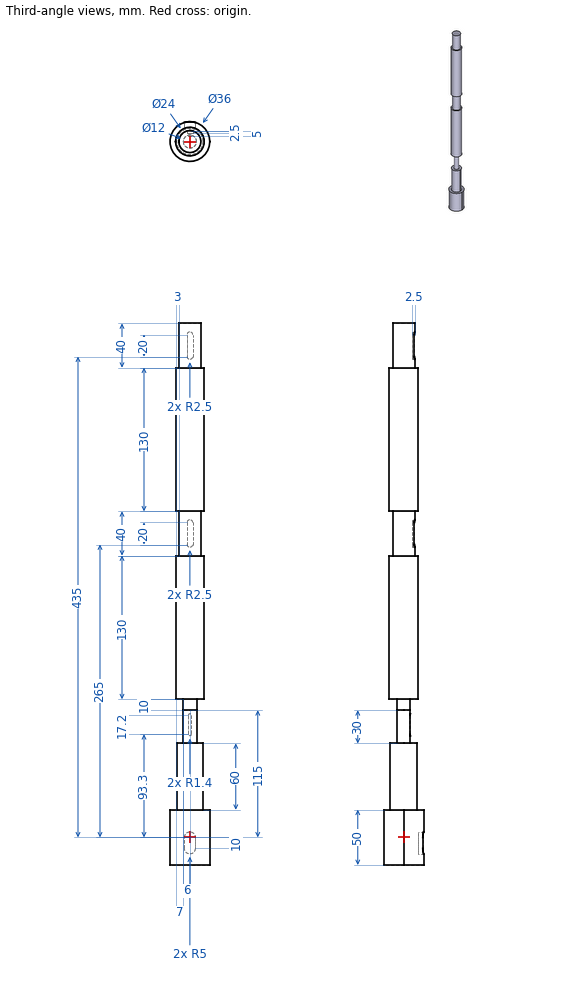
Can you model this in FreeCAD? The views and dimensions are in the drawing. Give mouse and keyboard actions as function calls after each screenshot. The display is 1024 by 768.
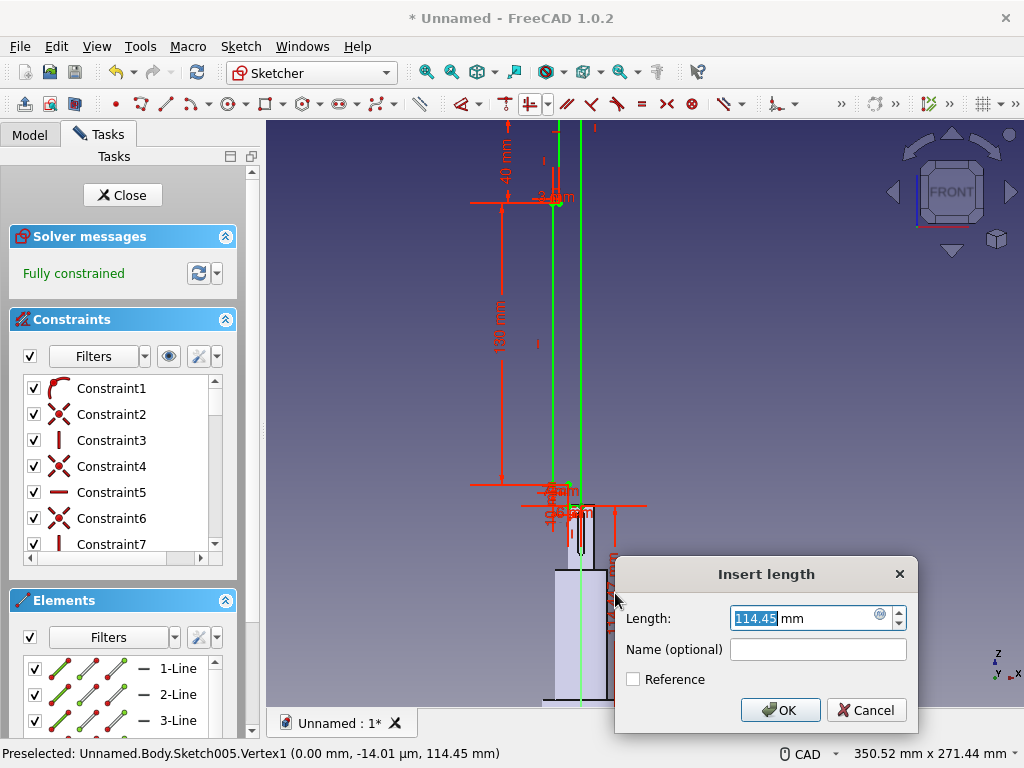
text(115)
key(Return)
key(Escape)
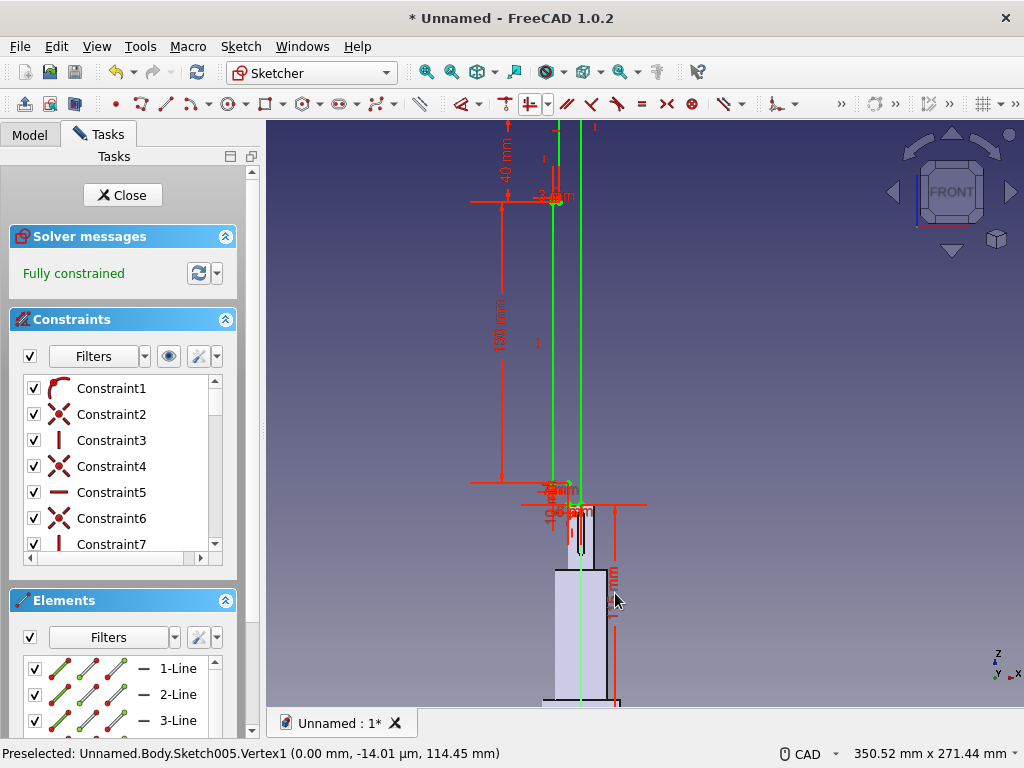
click(123, 195)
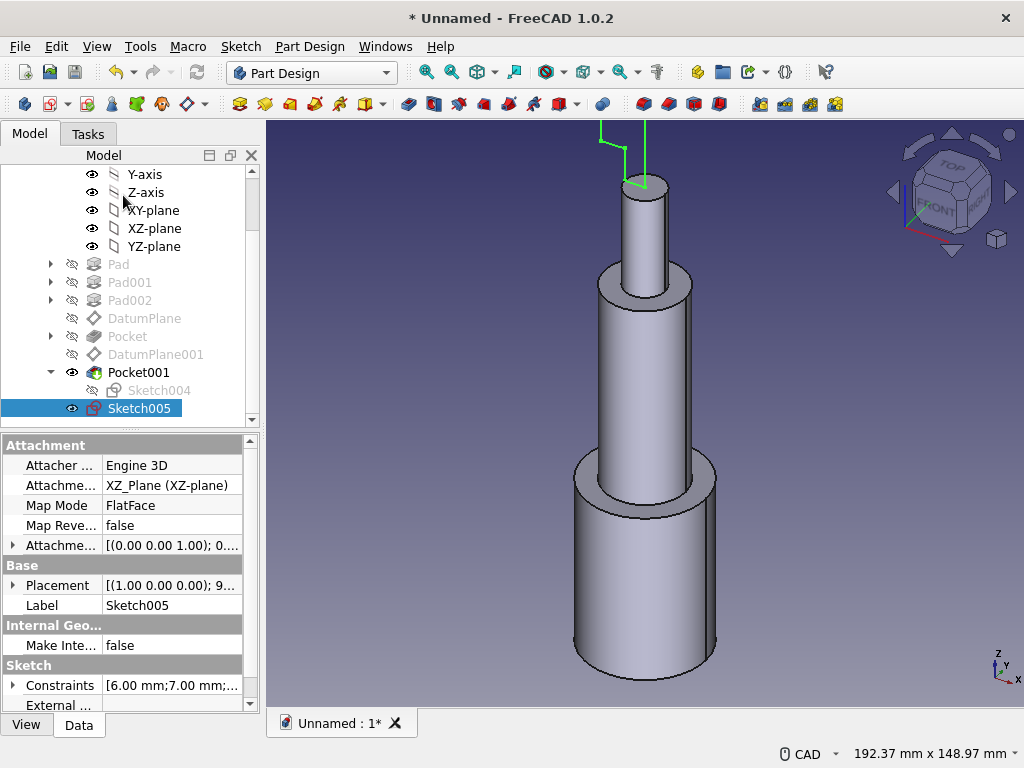
click(265, 104)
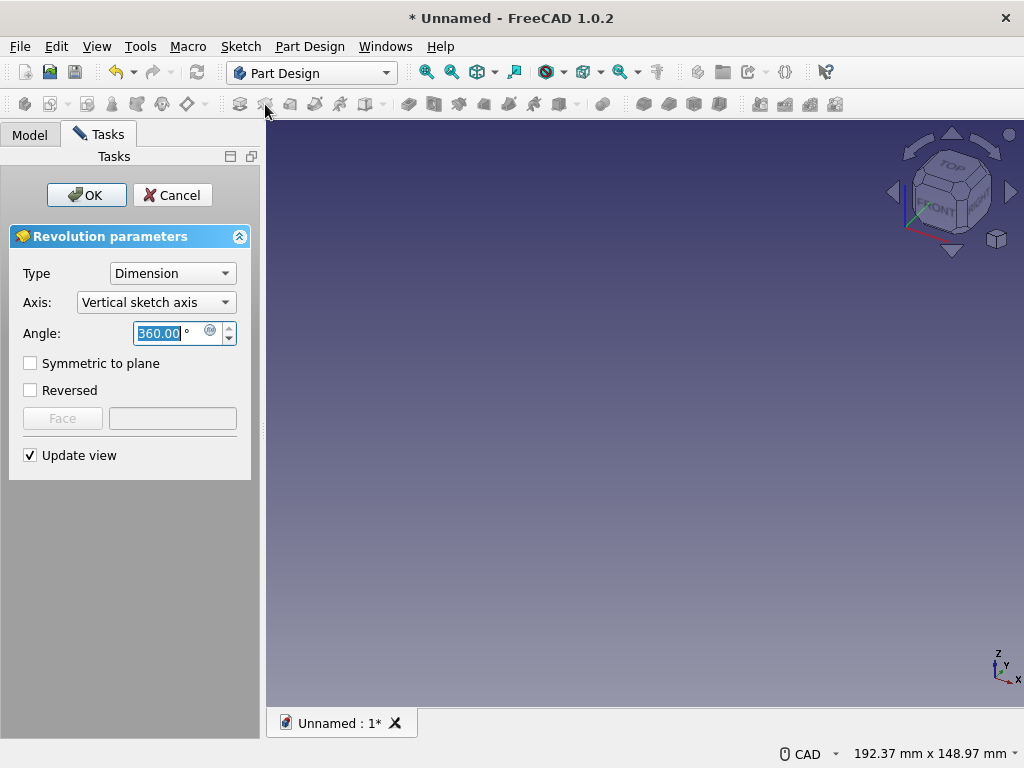
click(87, 195)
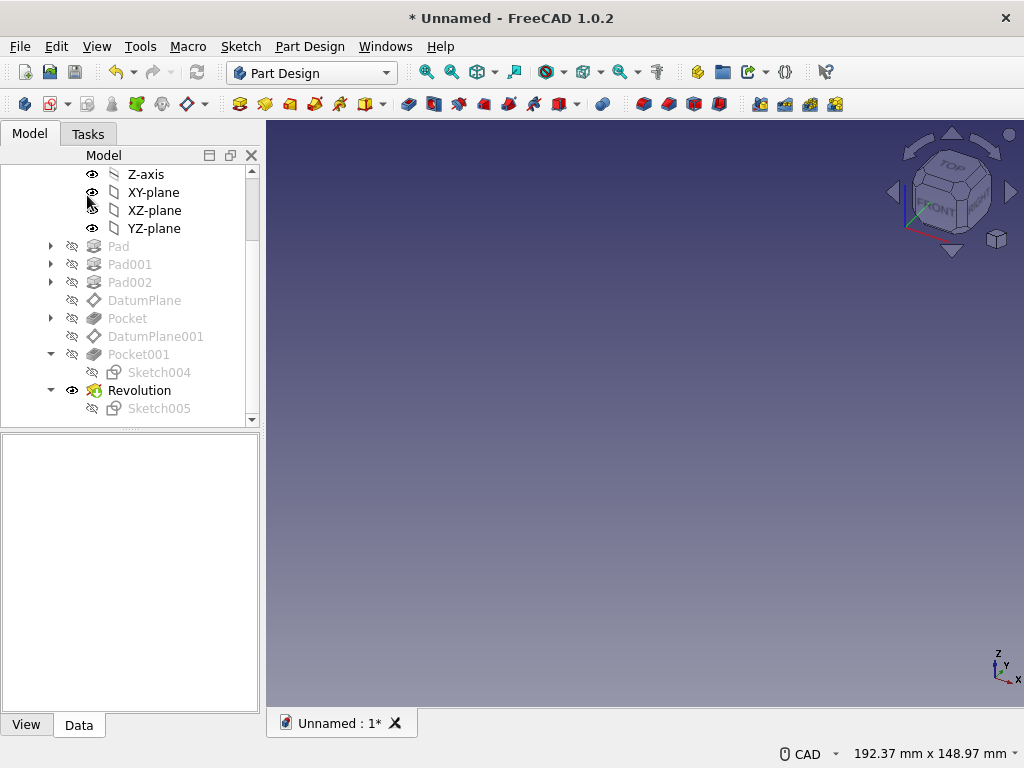
click(427, 72)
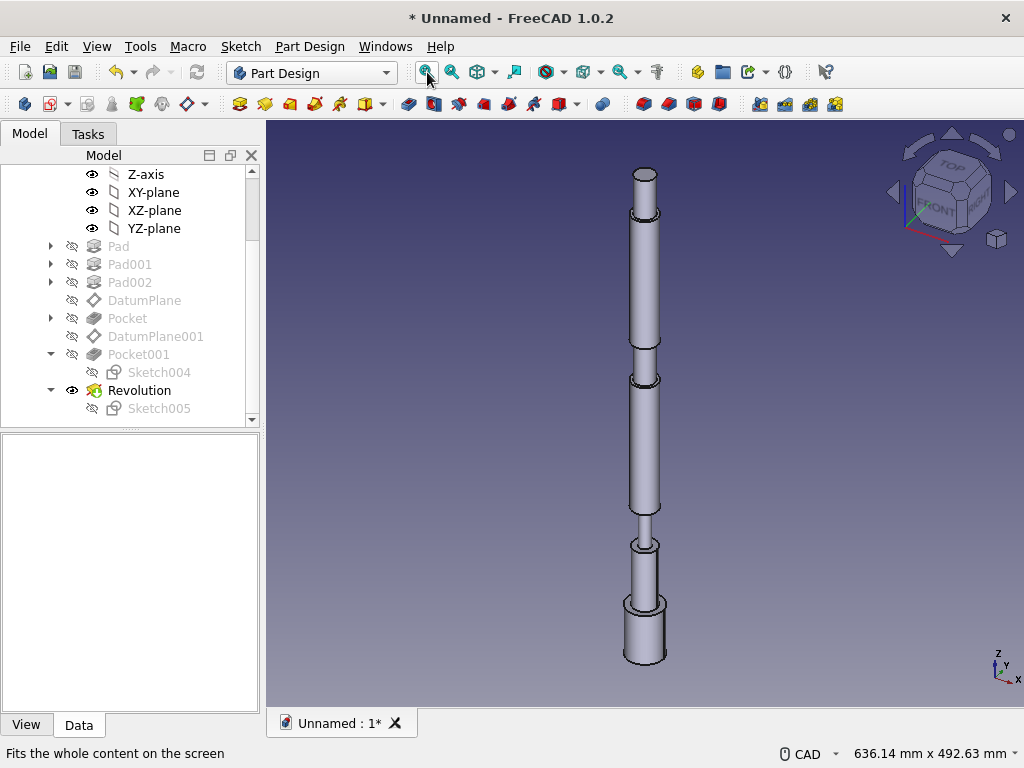
scroll(161, 296, down, 3)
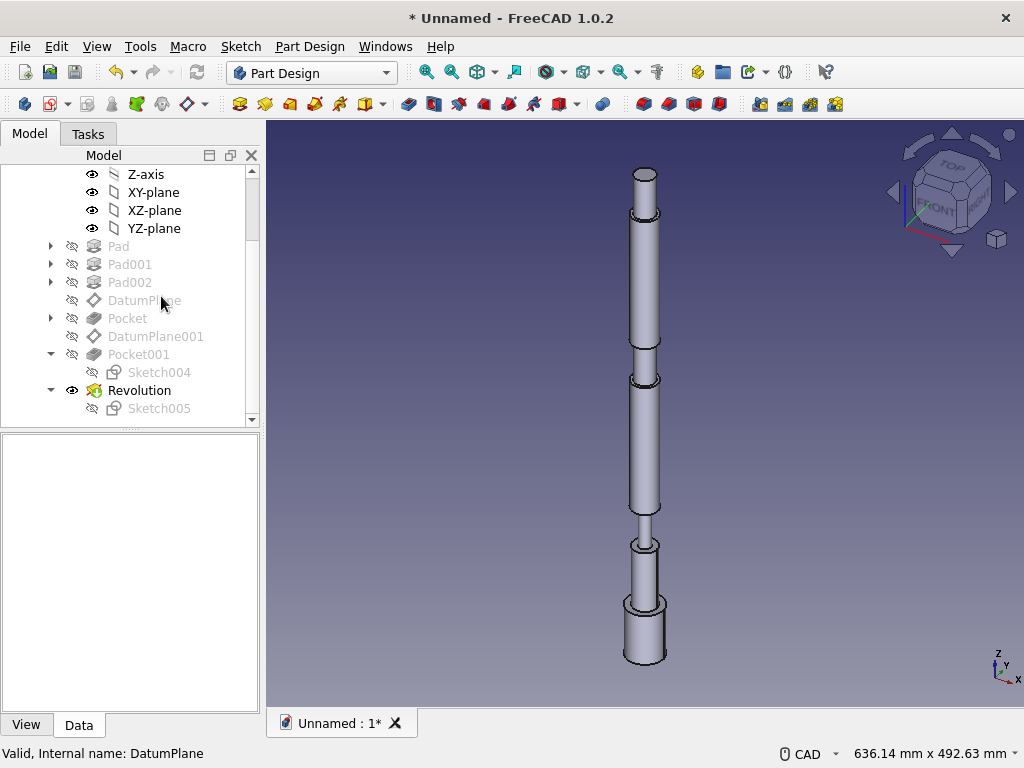
scroll(161, 296, up, 15)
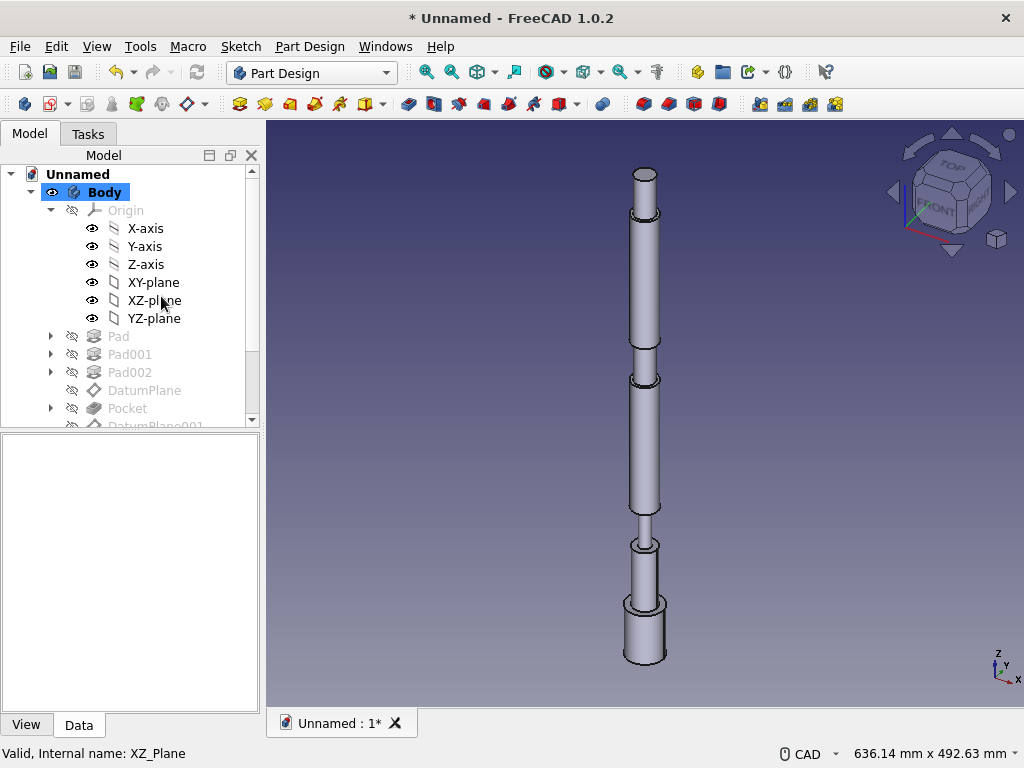
click(137, 300)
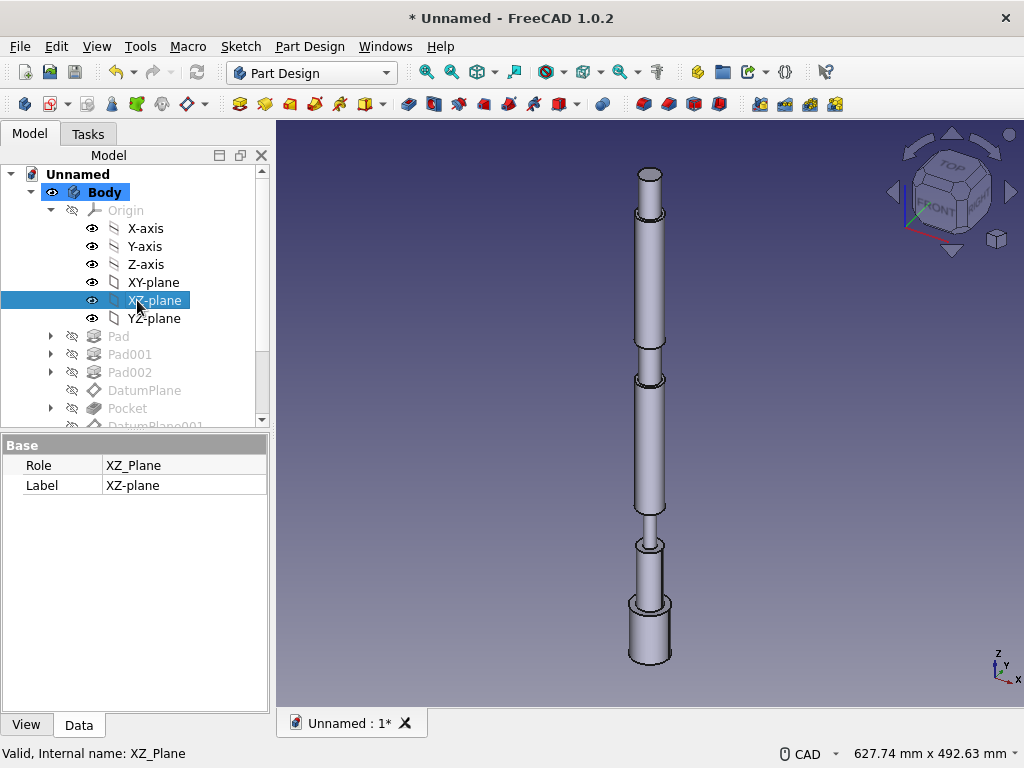
click(186, 104)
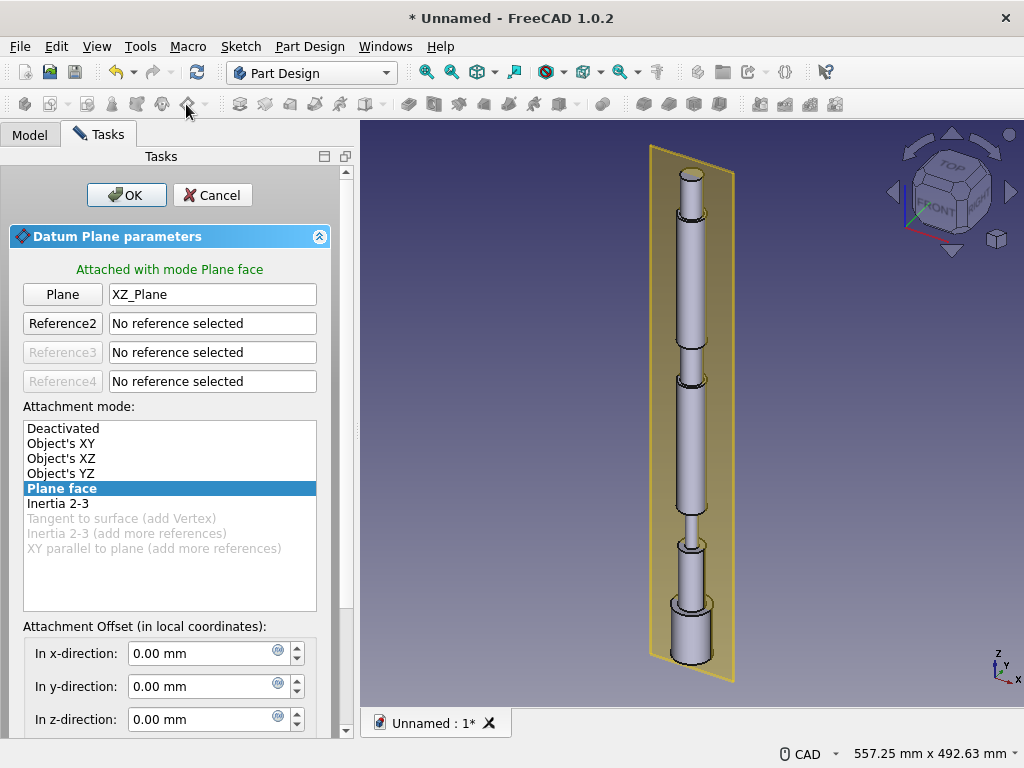
triple_click(210, 720)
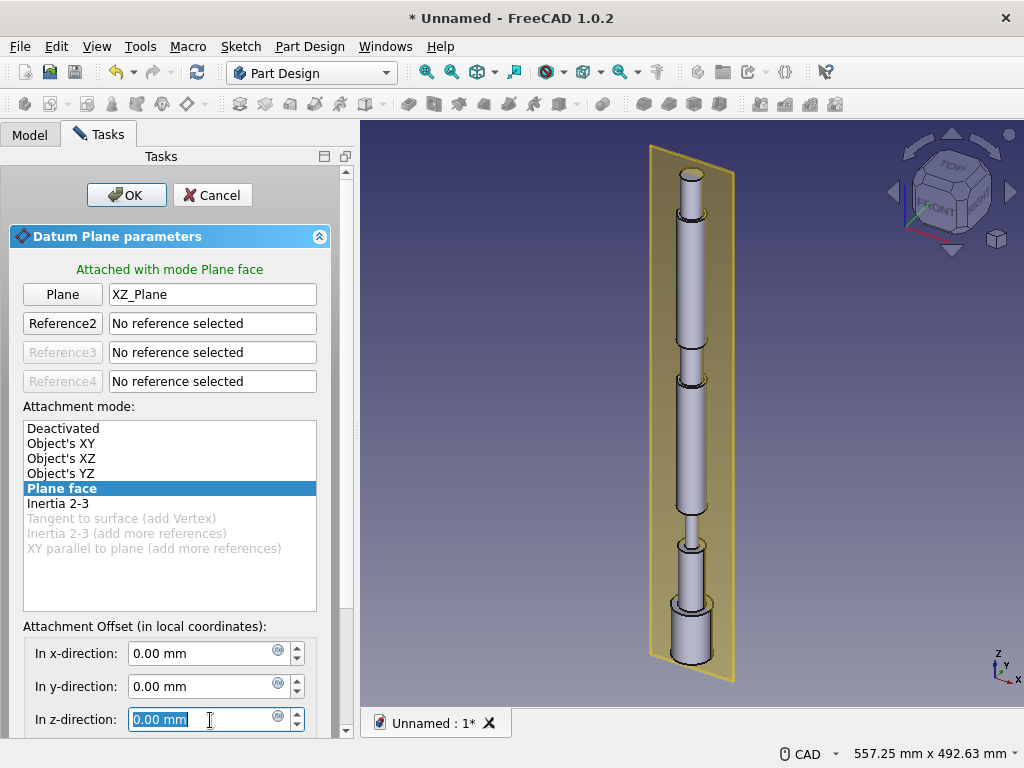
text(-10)
key(Tab)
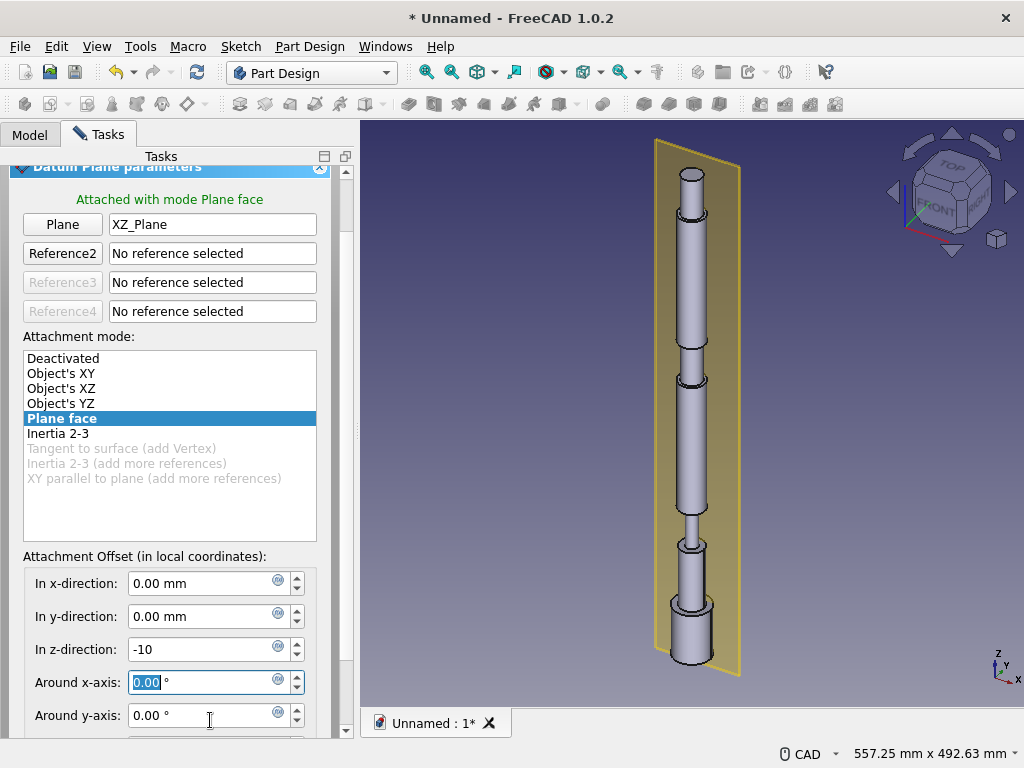
scroll(346, 452, up, 2)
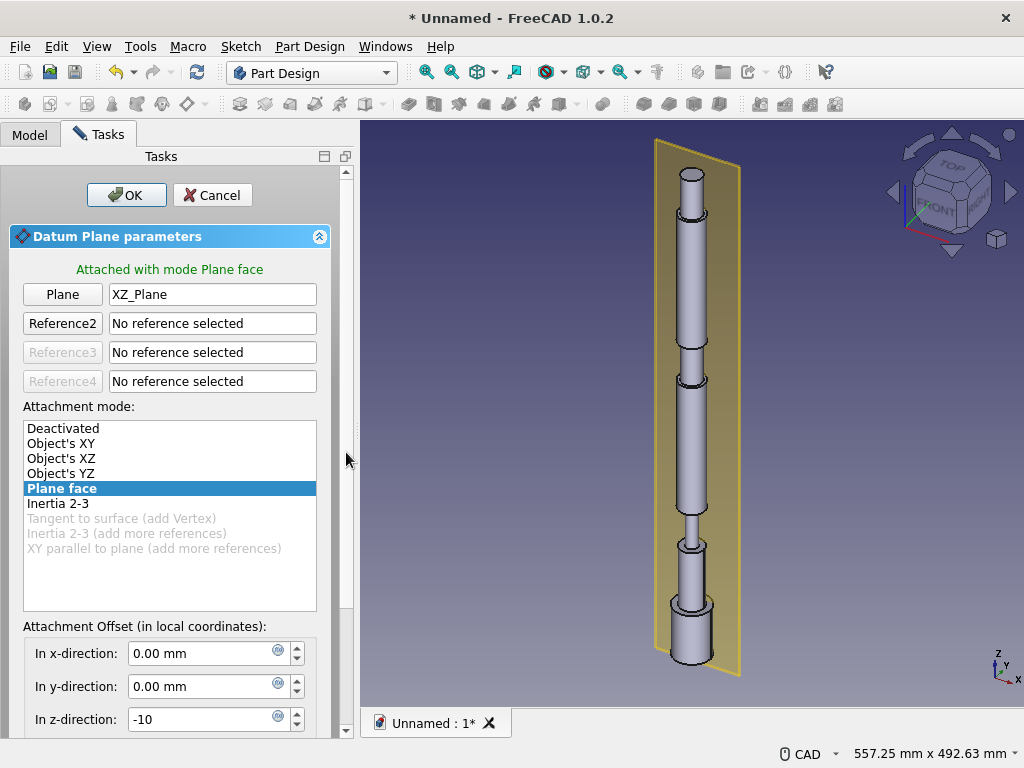
click(127, 195)